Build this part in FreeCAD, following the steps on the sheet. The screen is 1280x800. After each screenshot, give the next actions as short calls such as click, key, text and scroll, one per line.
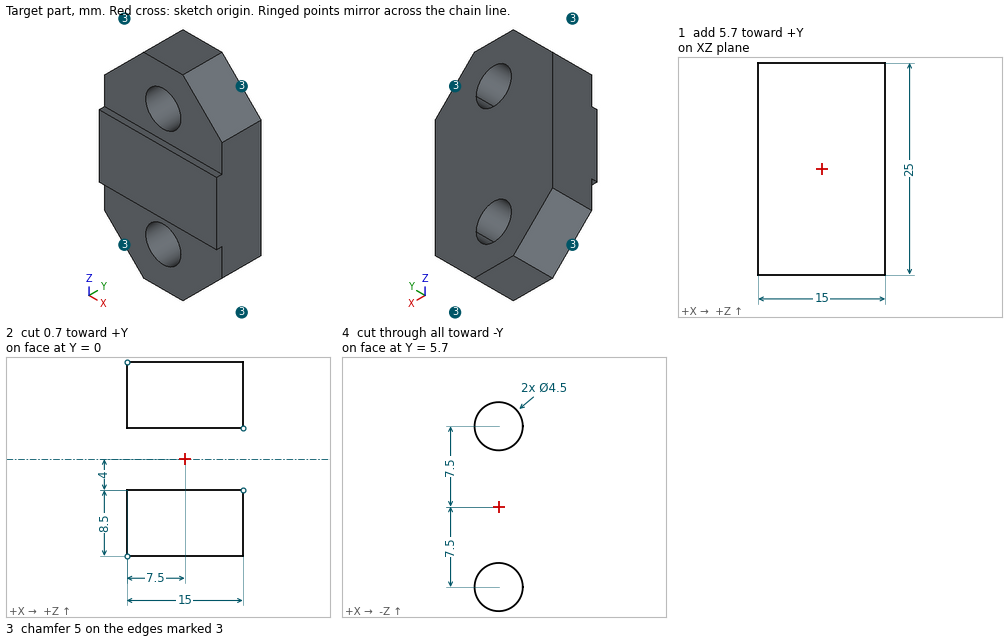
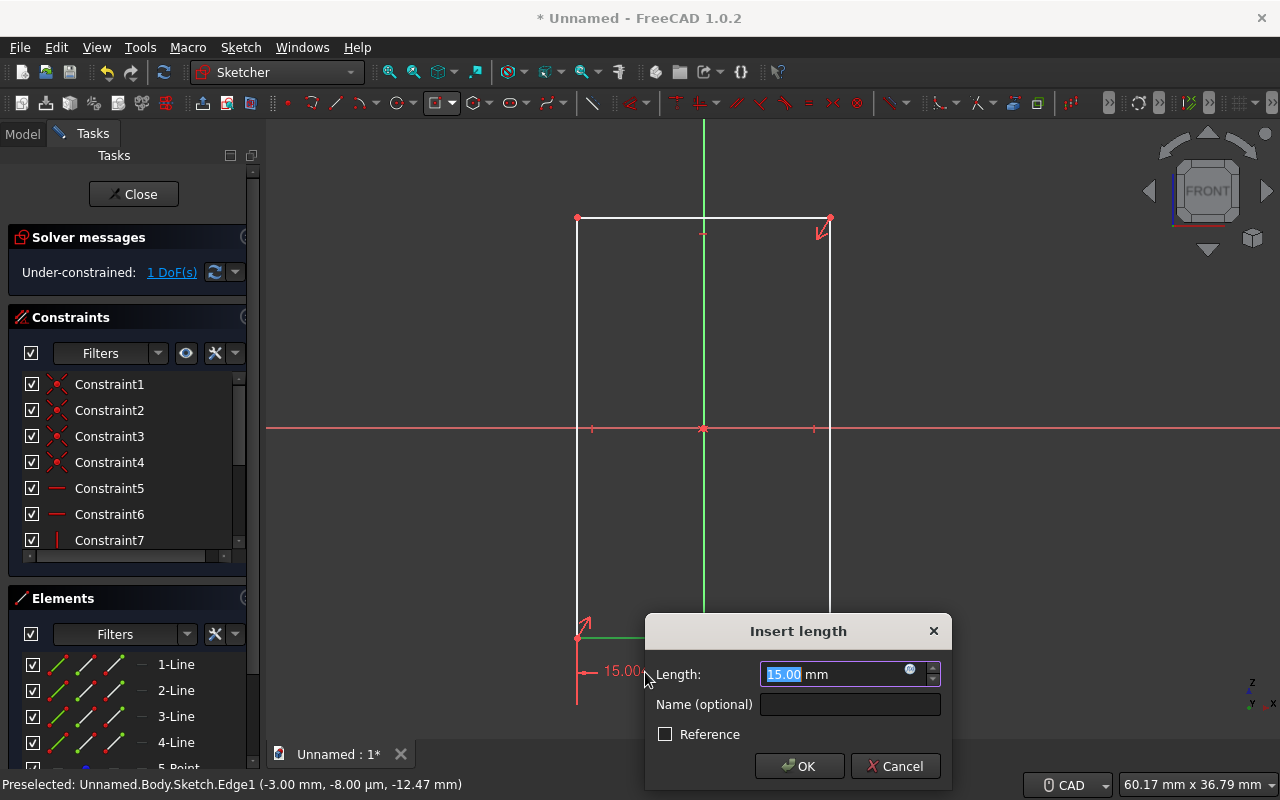
text(15)
key(Return)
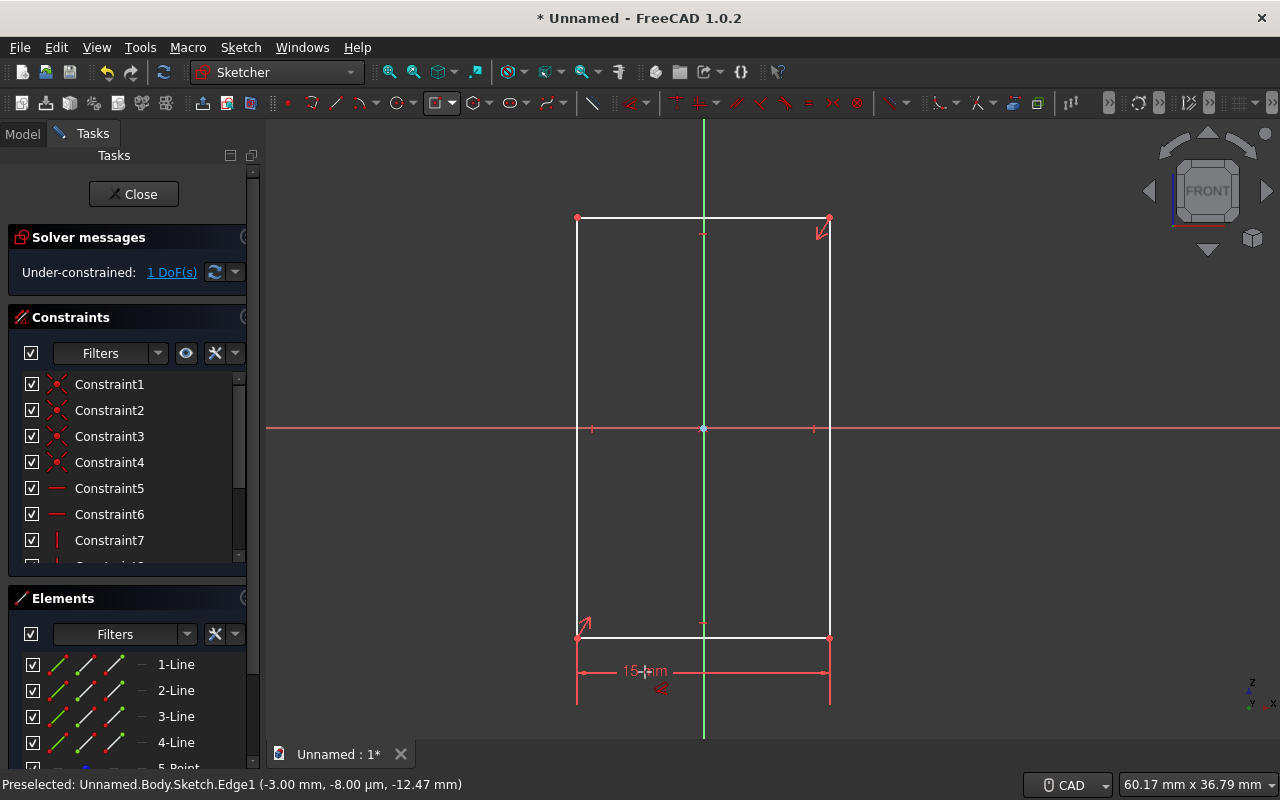
click(830, 512)
click(864, 331)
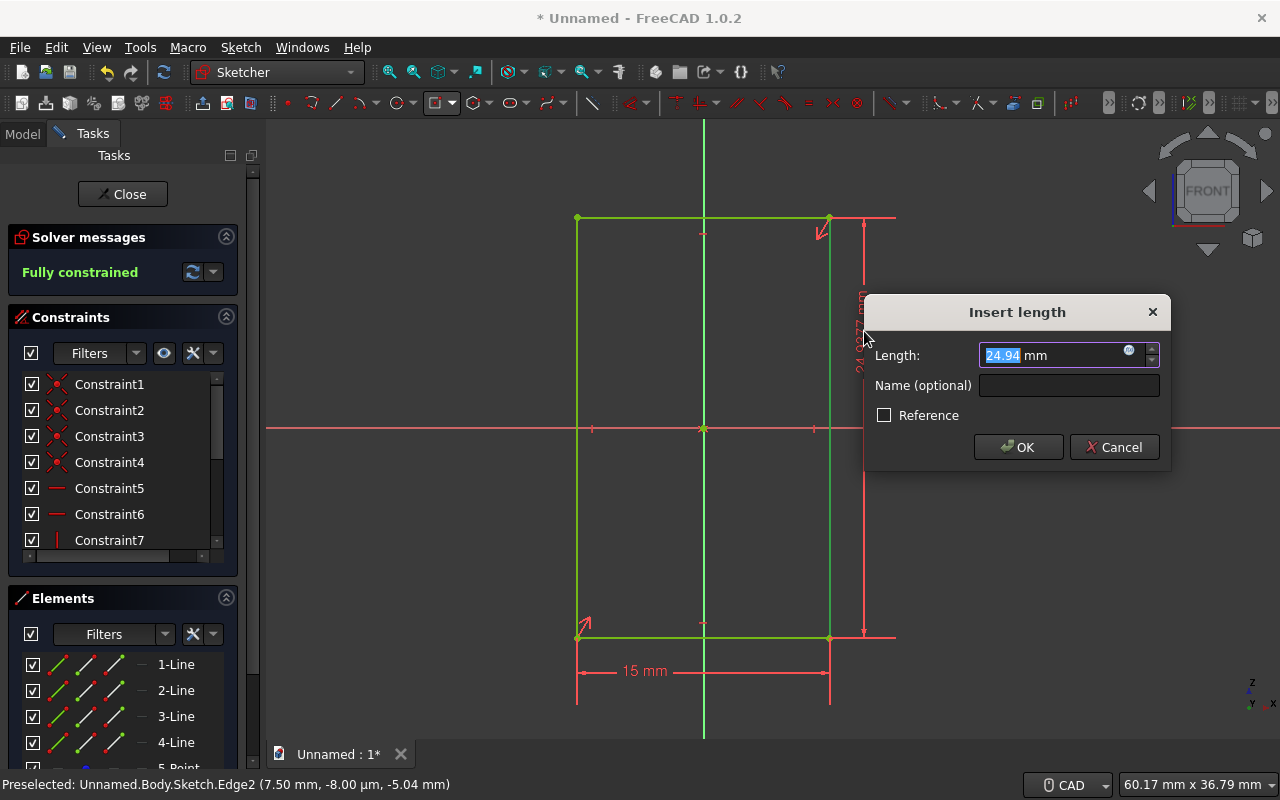
text(25)
key(Return)
key(Escape)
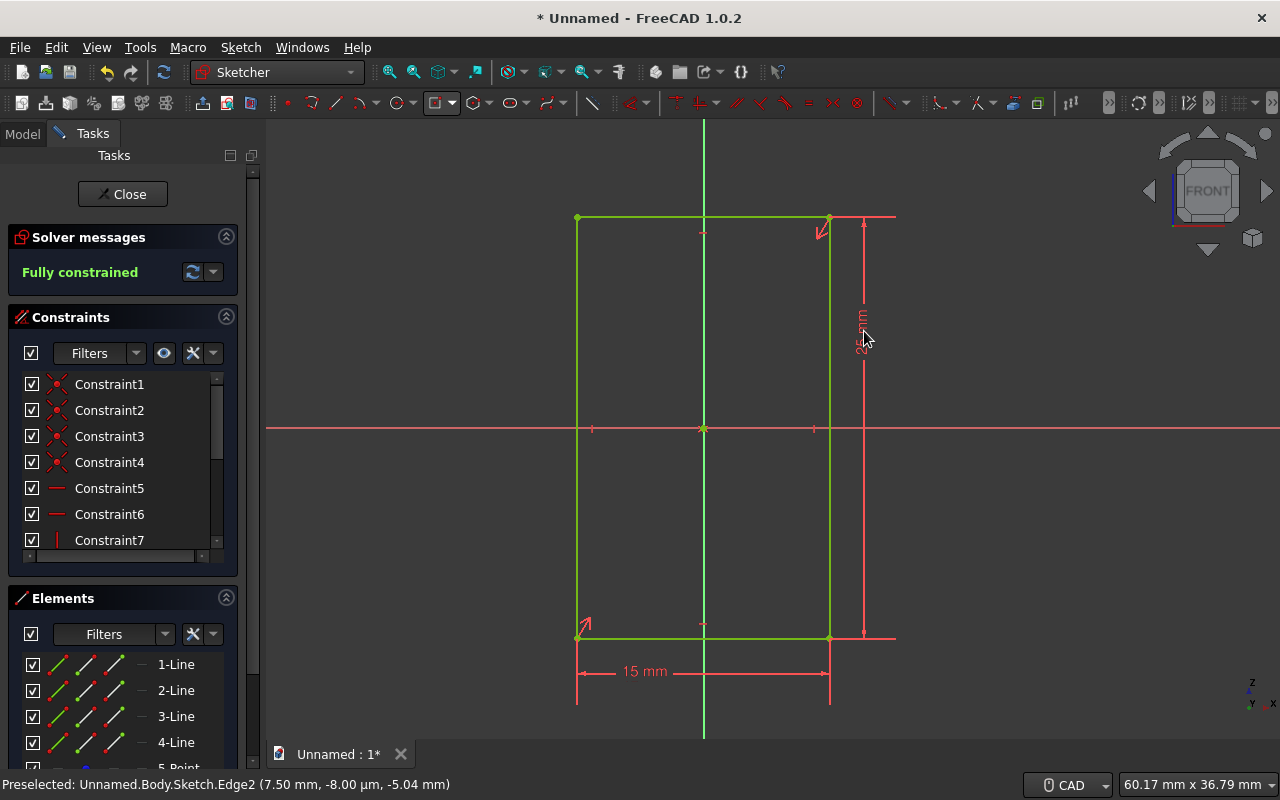
click(123, 194)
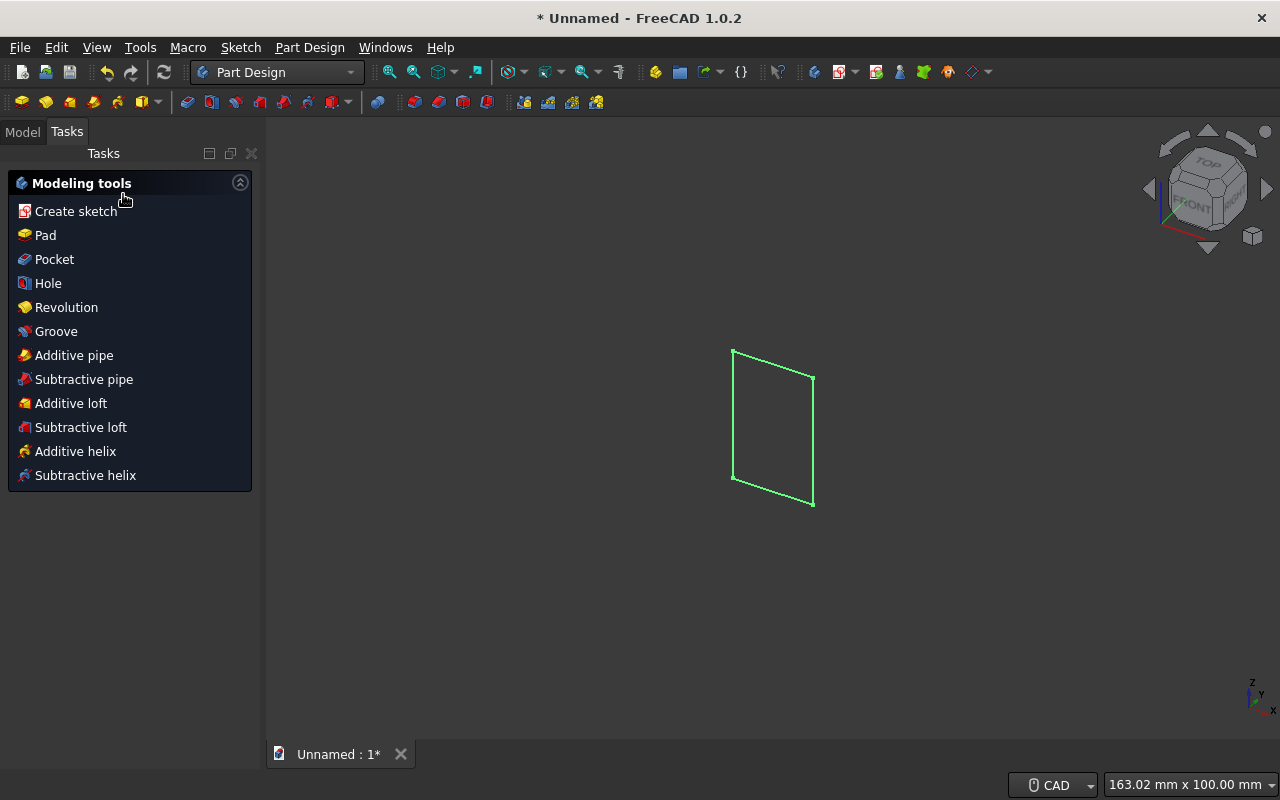
click(22, 102)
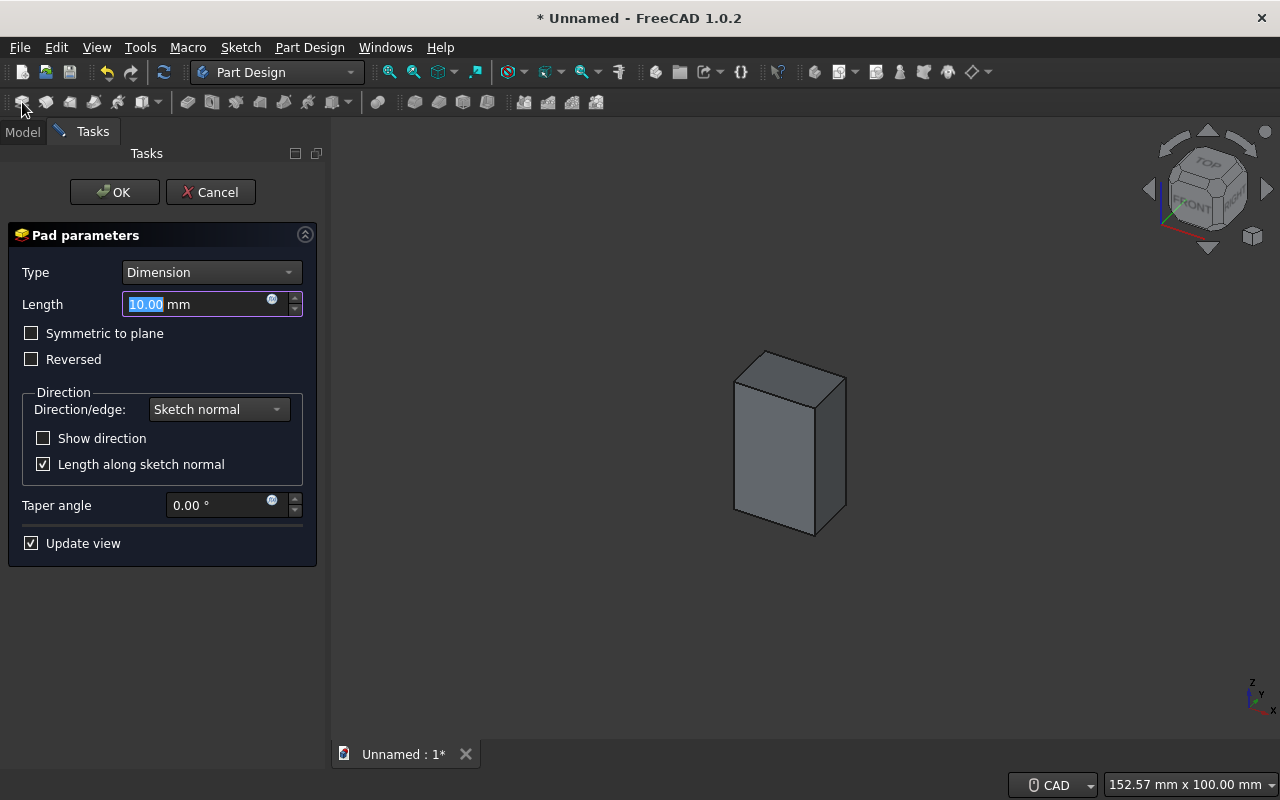
text(5.7)
key(Tab)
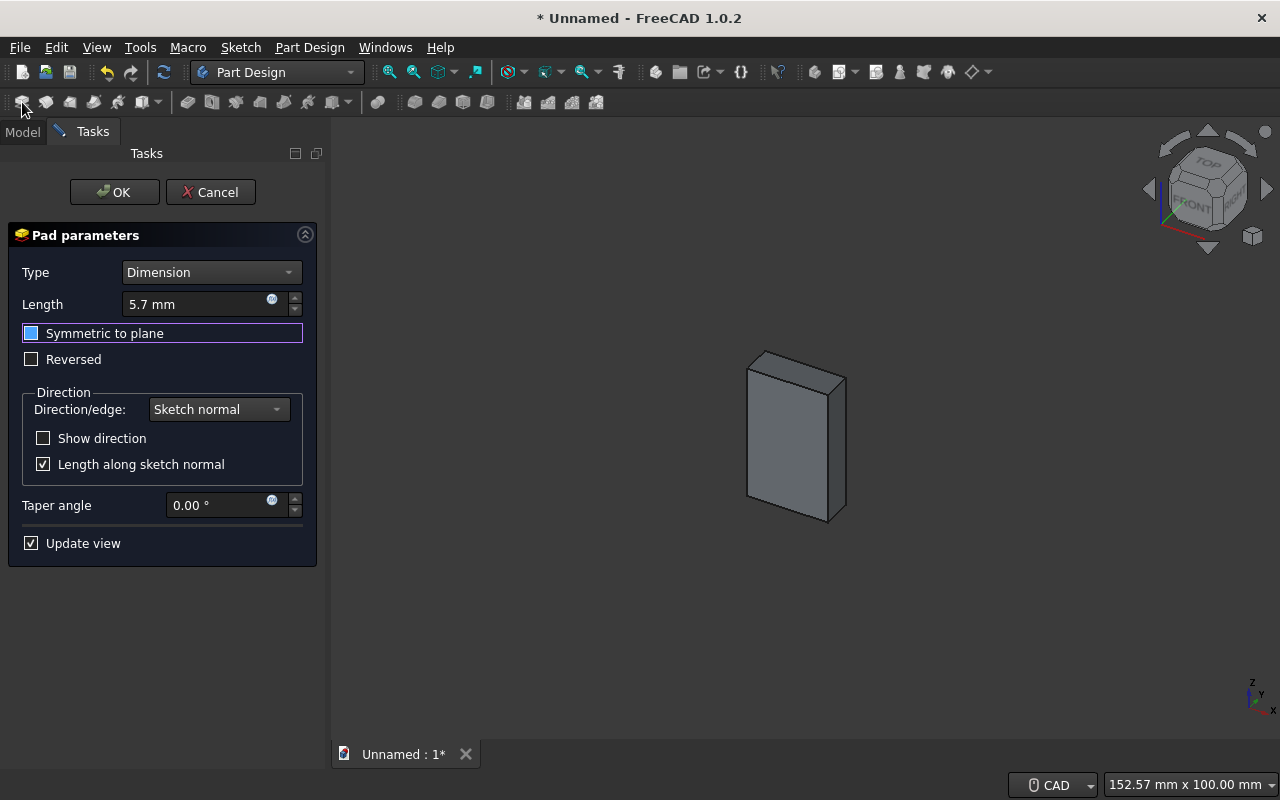
click(30, 359)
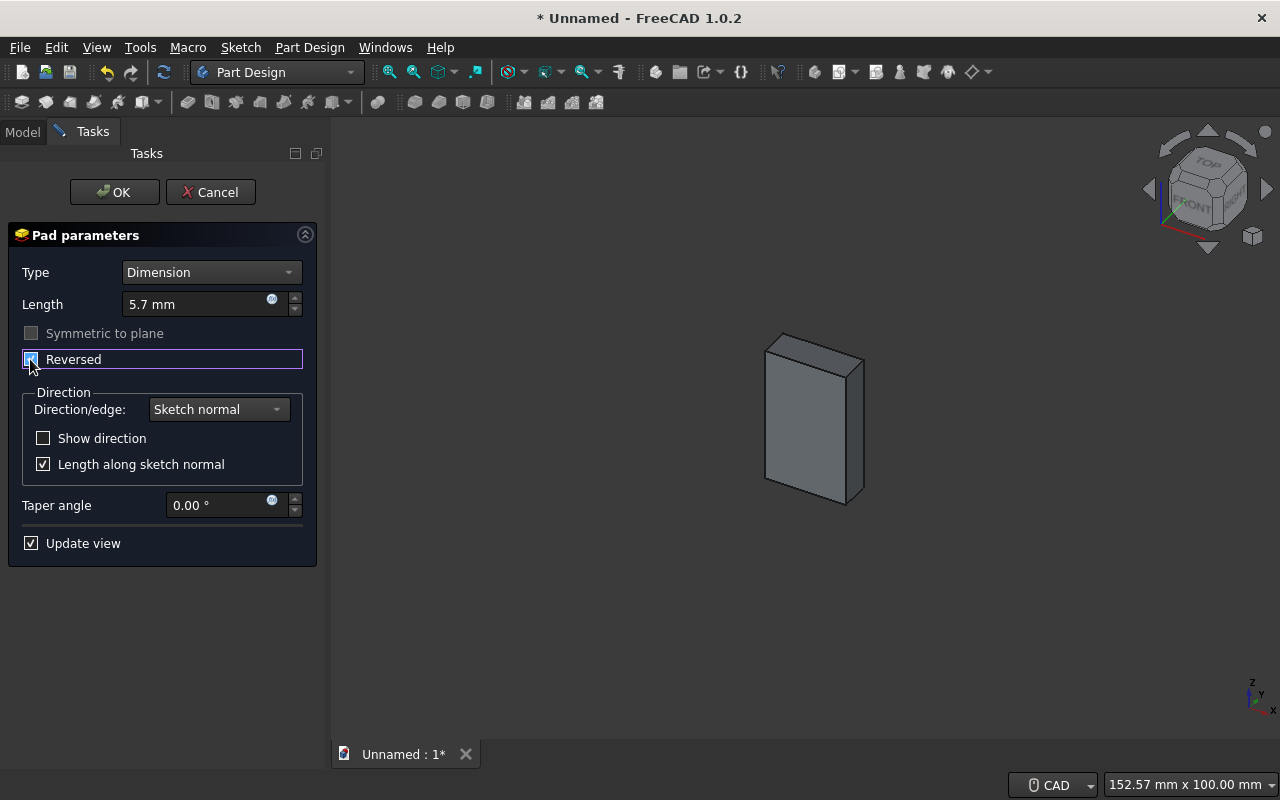
click(115, 192)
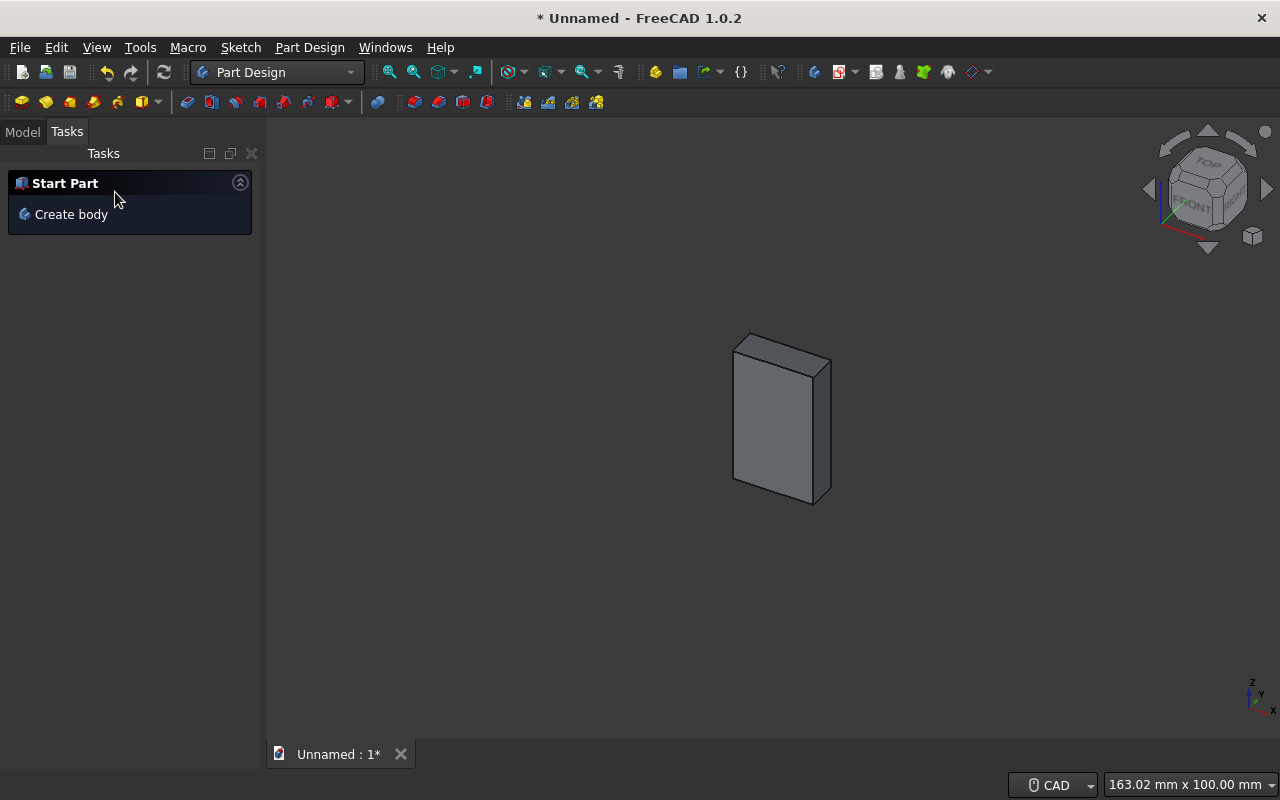
key(v)
key(f)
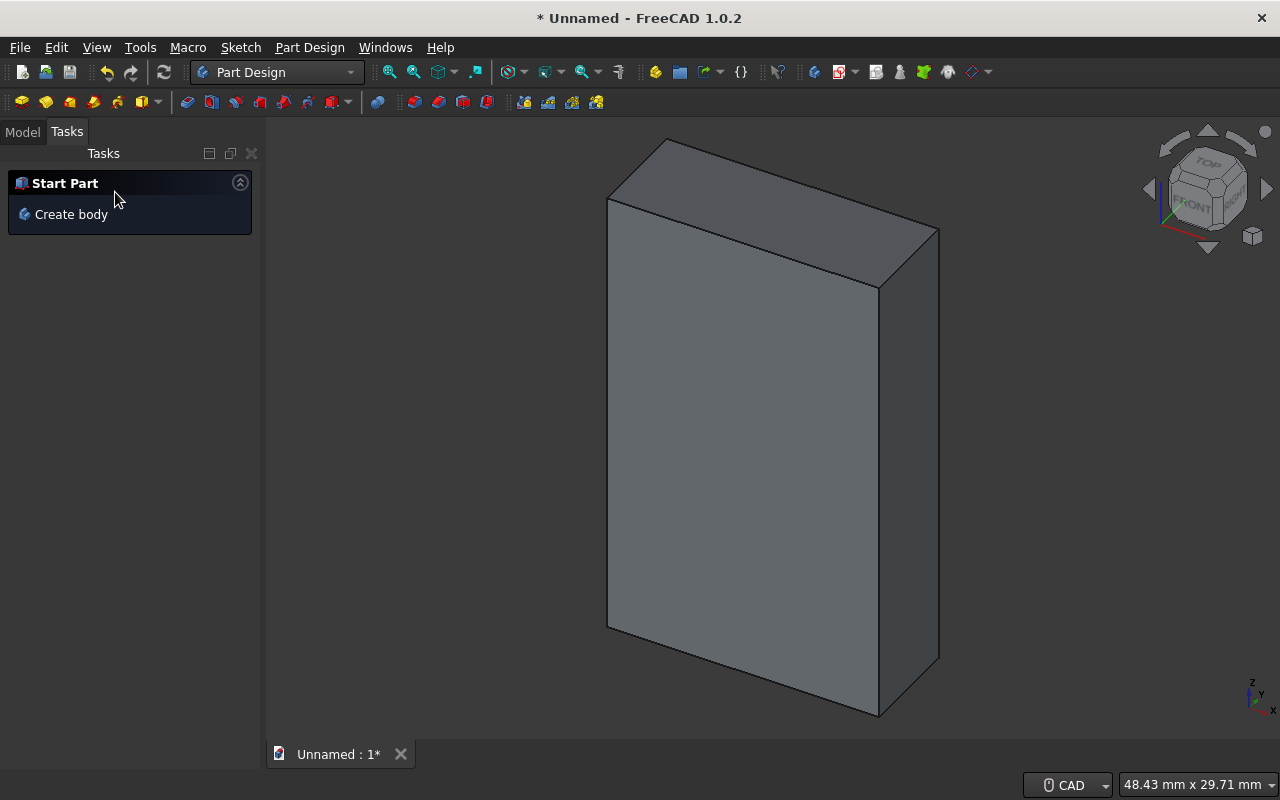
click(743, 395)